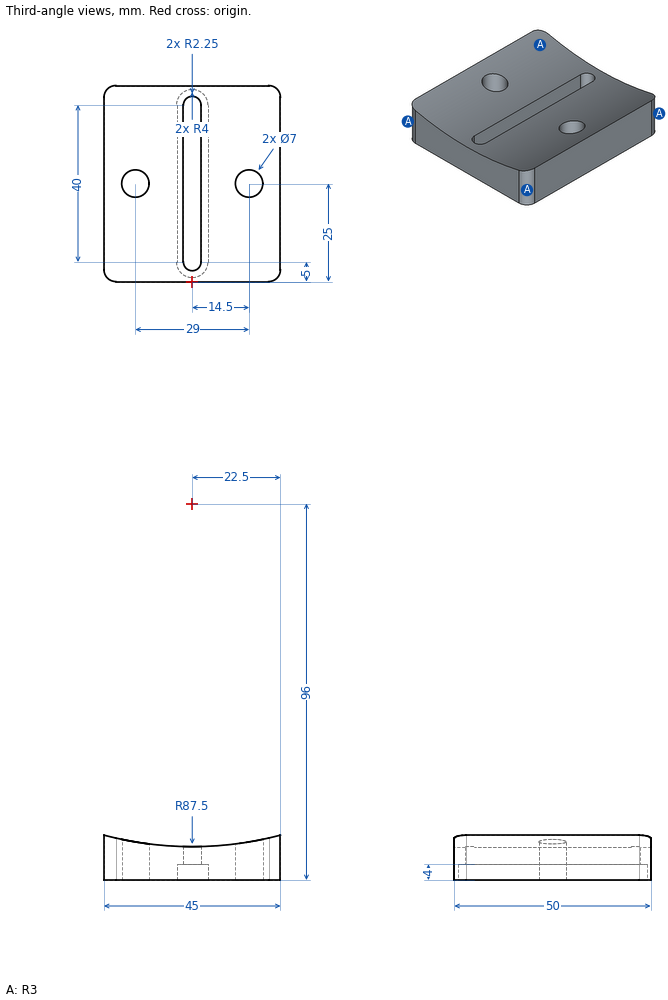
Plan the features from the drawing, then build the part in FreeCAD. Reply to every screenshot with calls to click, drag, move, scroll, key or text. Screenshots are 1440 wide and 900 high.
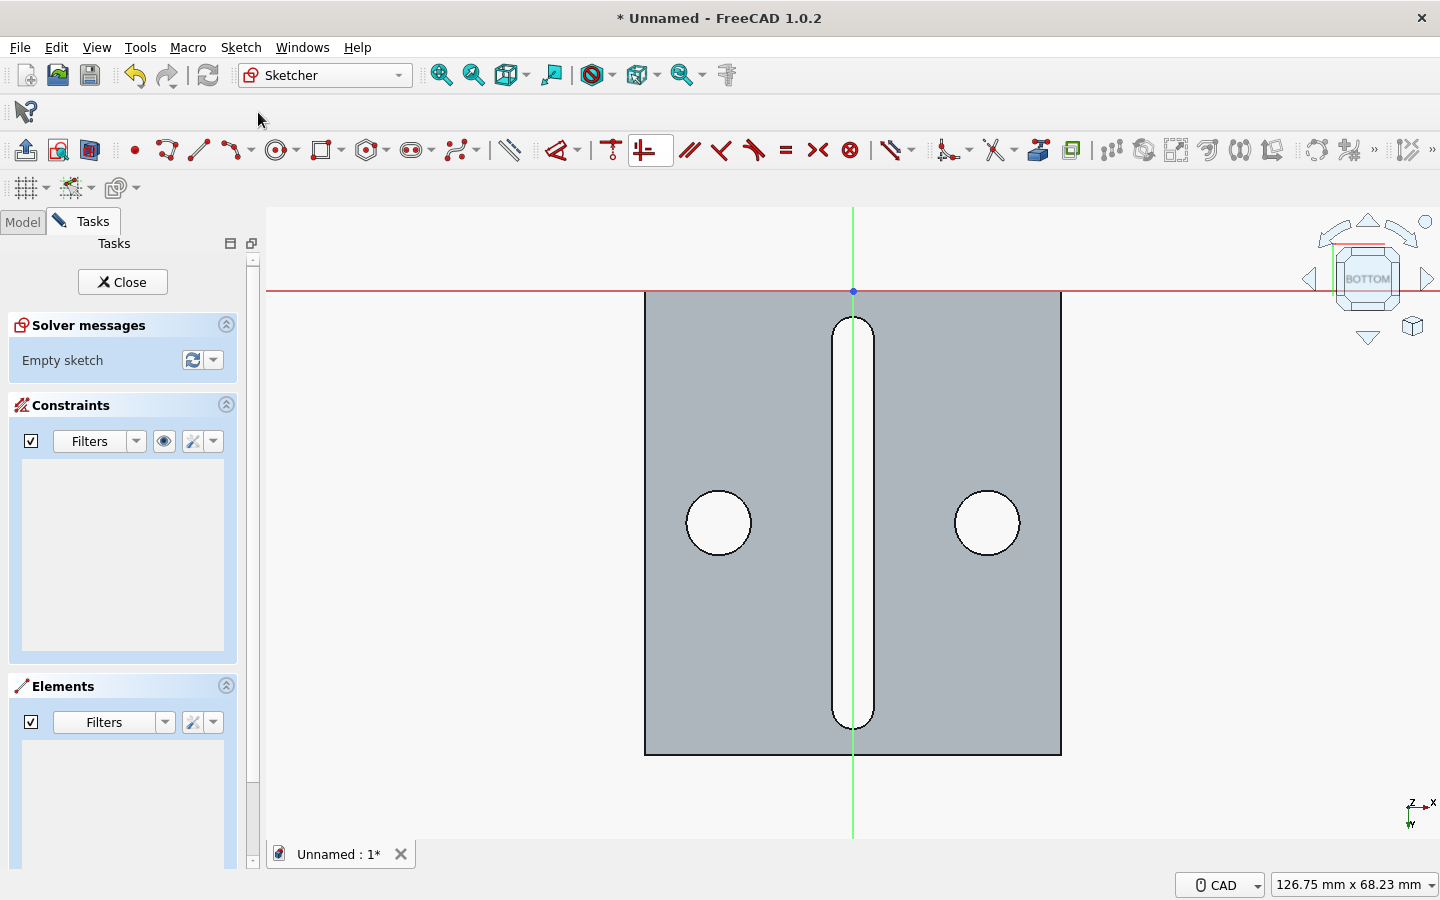
click(412, 150)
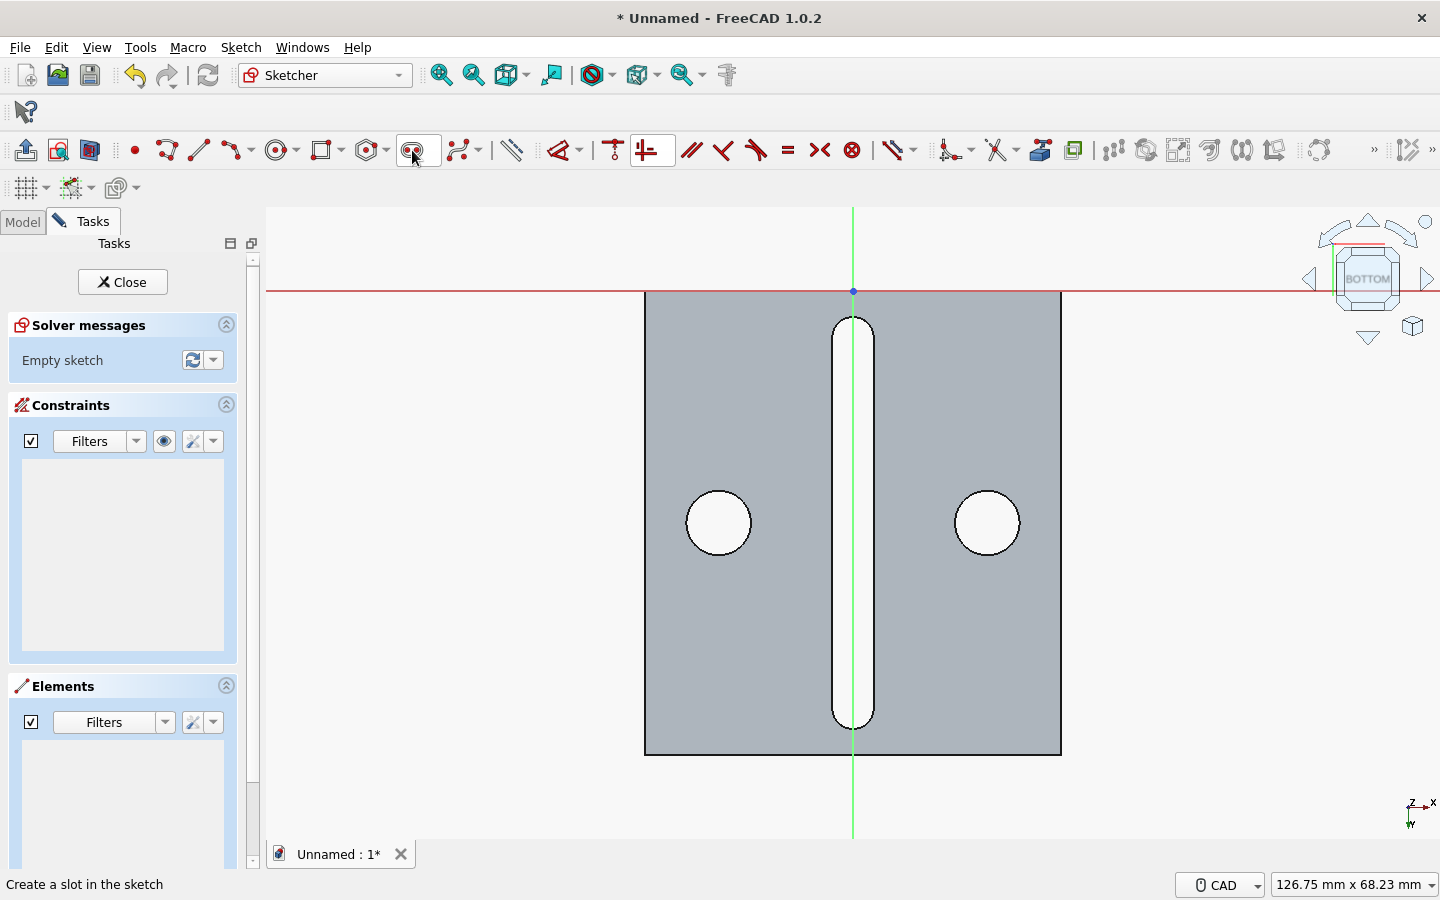
click(853, 708)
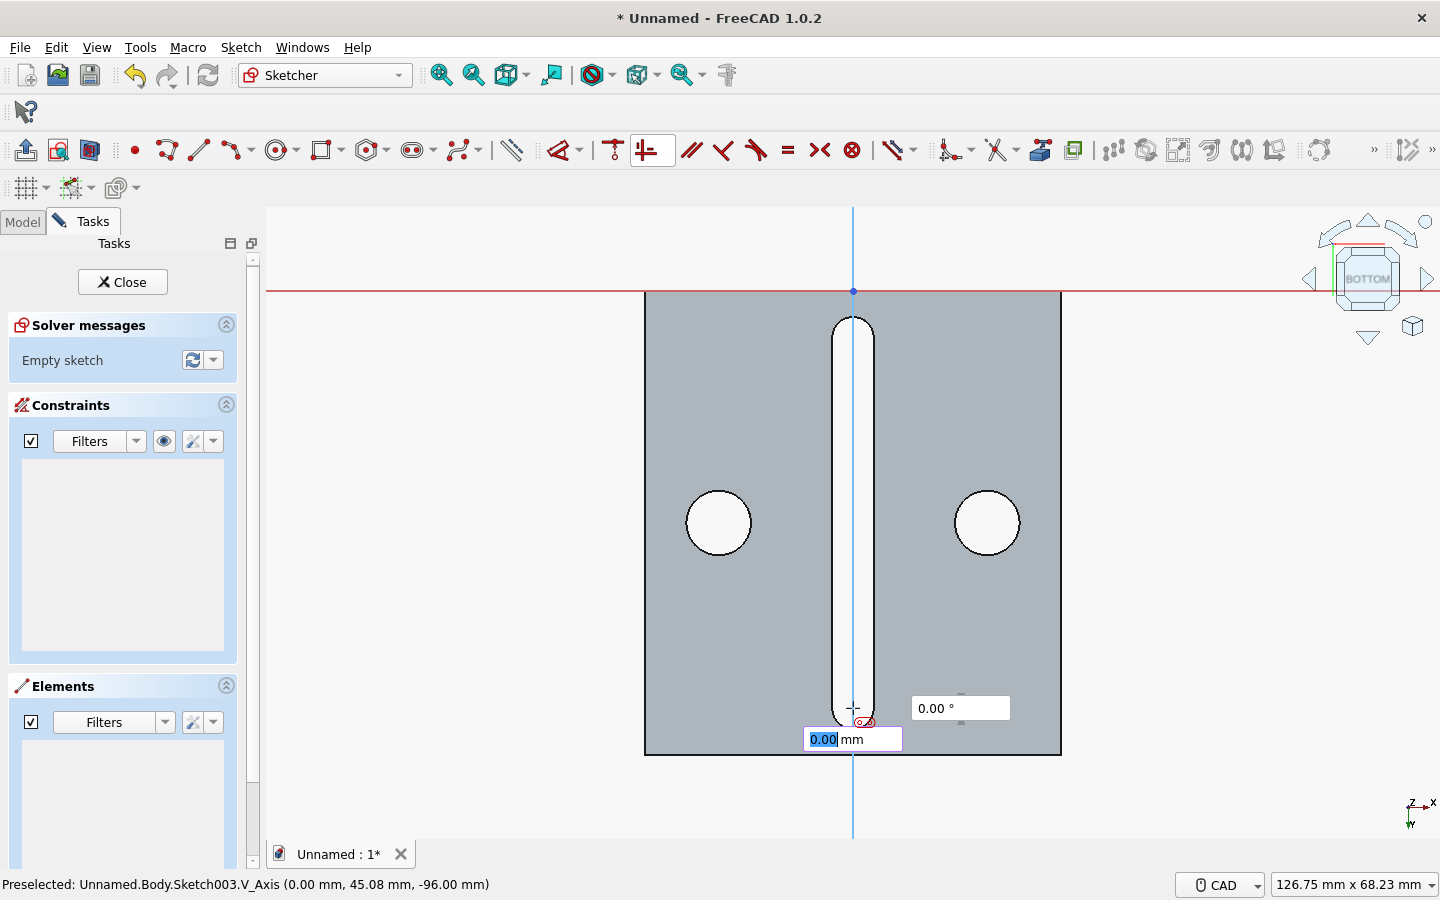
click(862, 338)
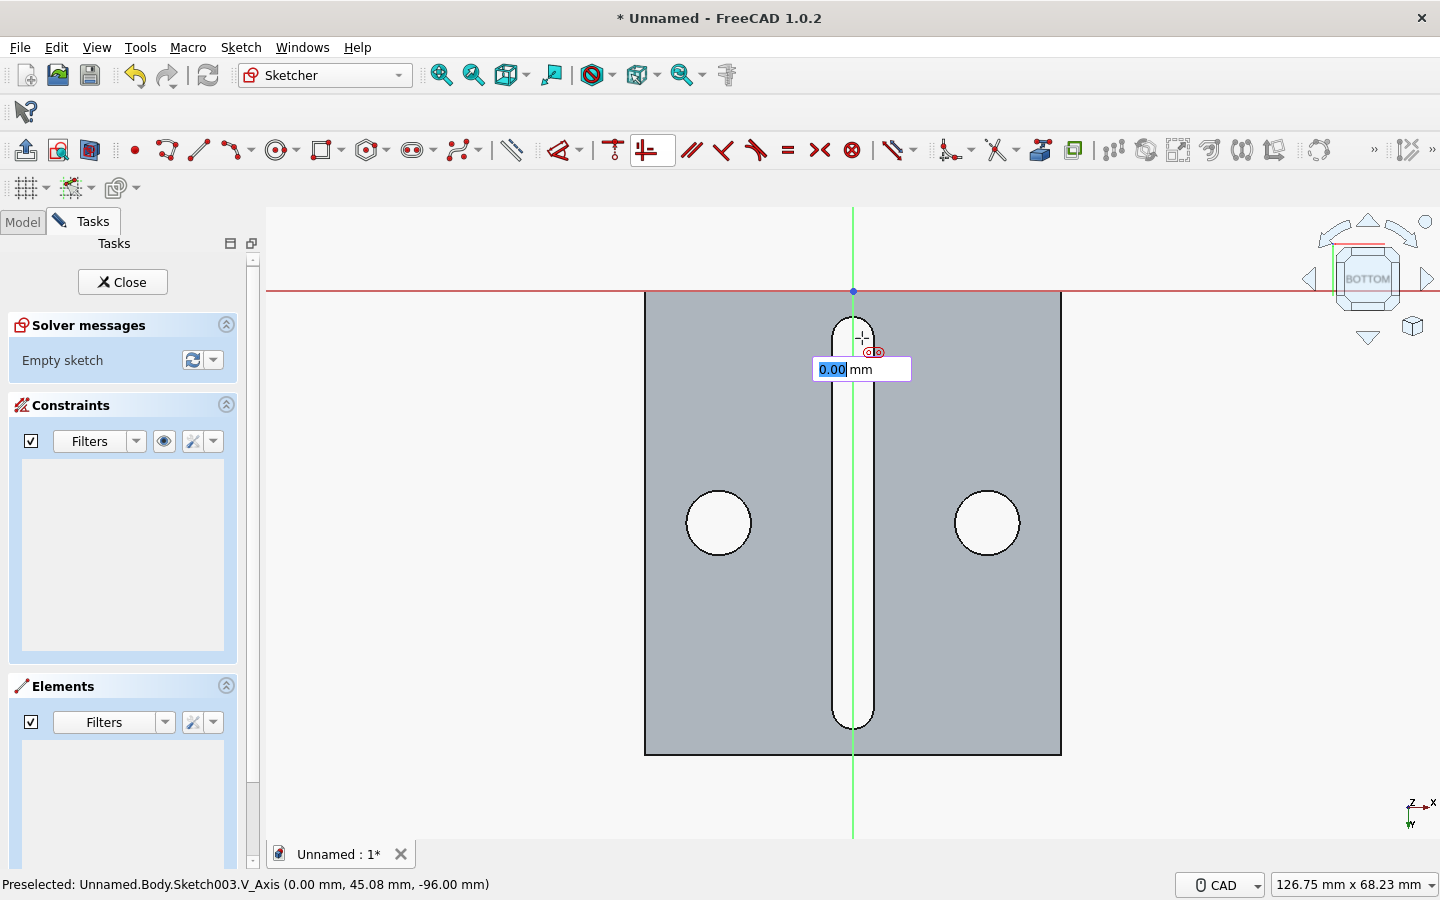
click(816, 523)
key(Escape)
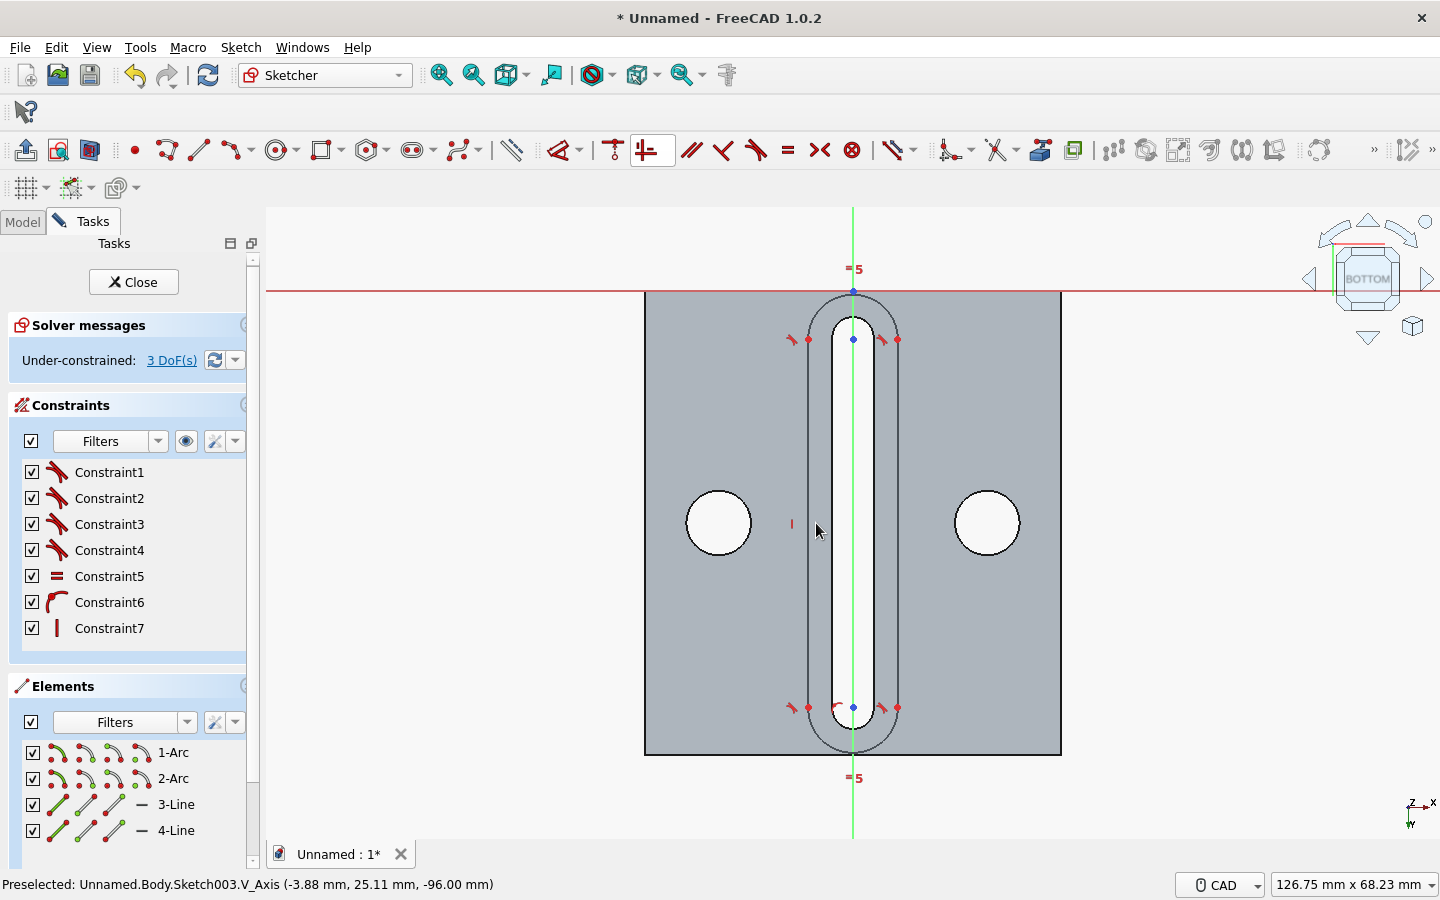
key(d)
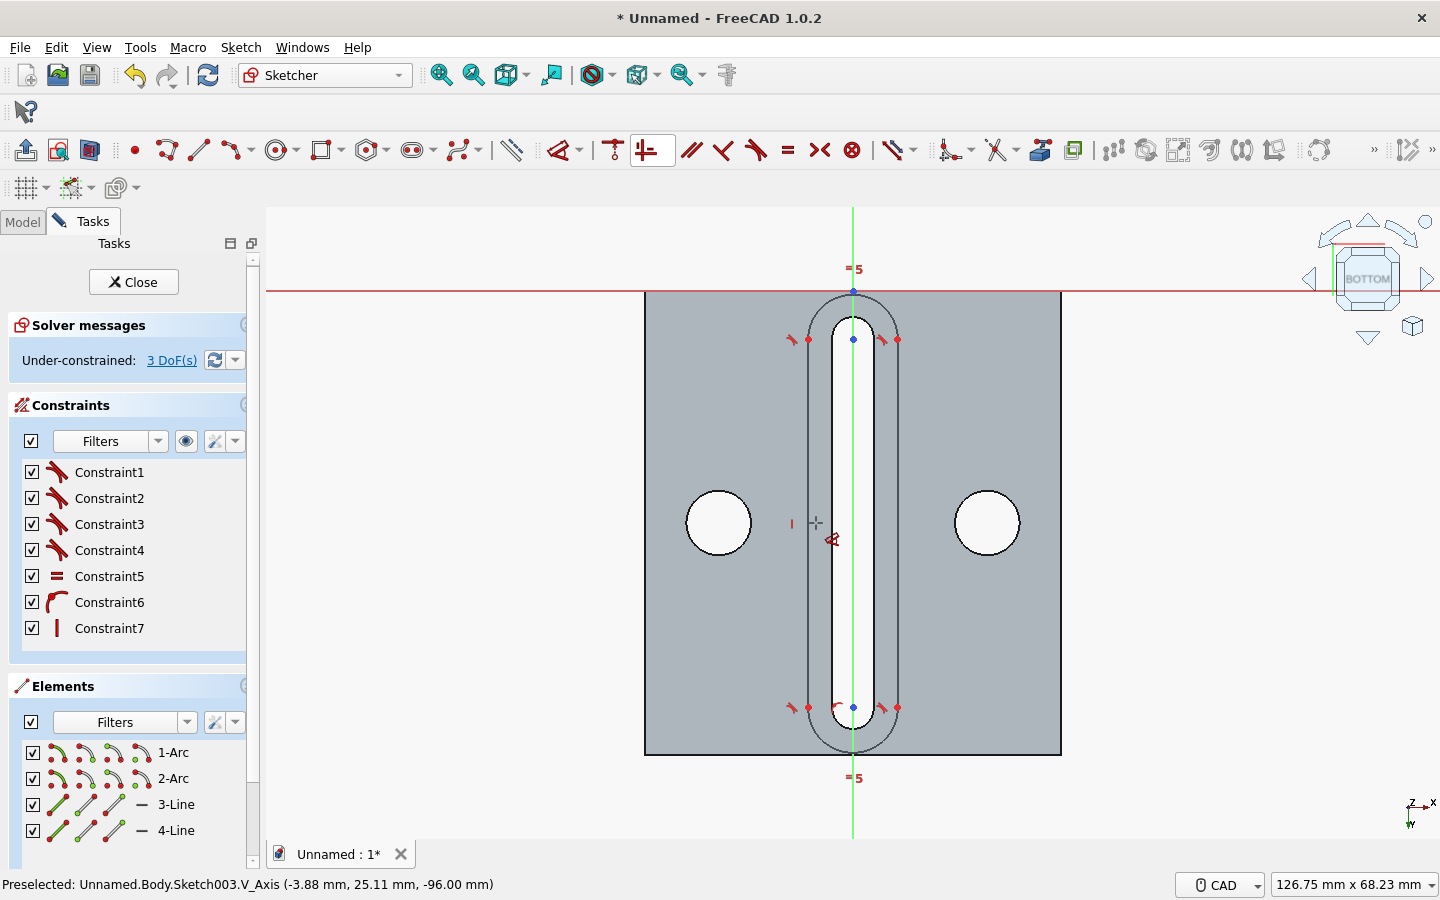
click(827, 744)
click(808, 770)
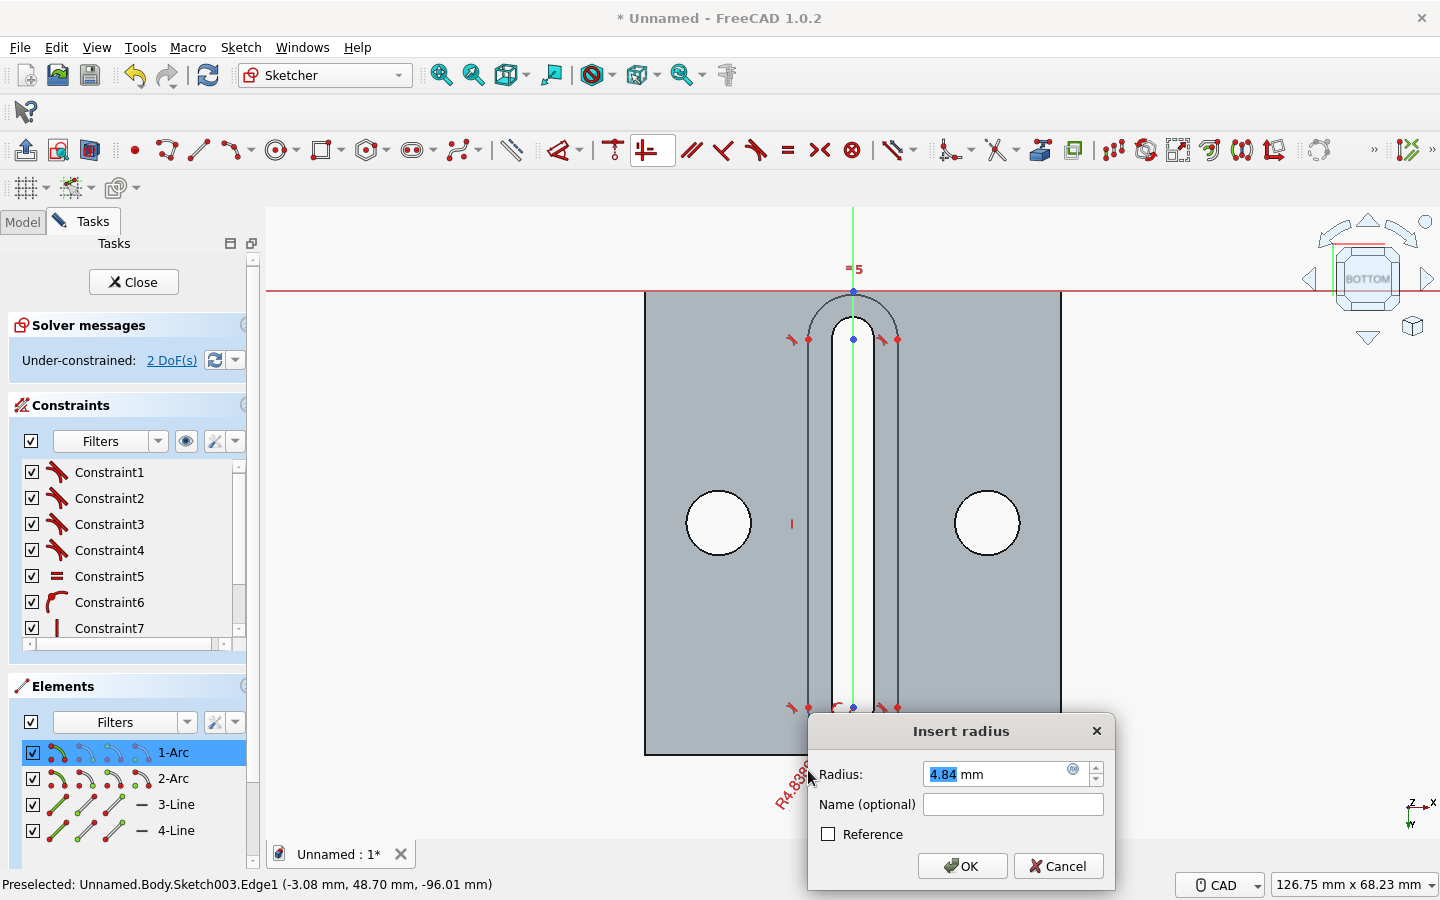
text(4)
key(Return)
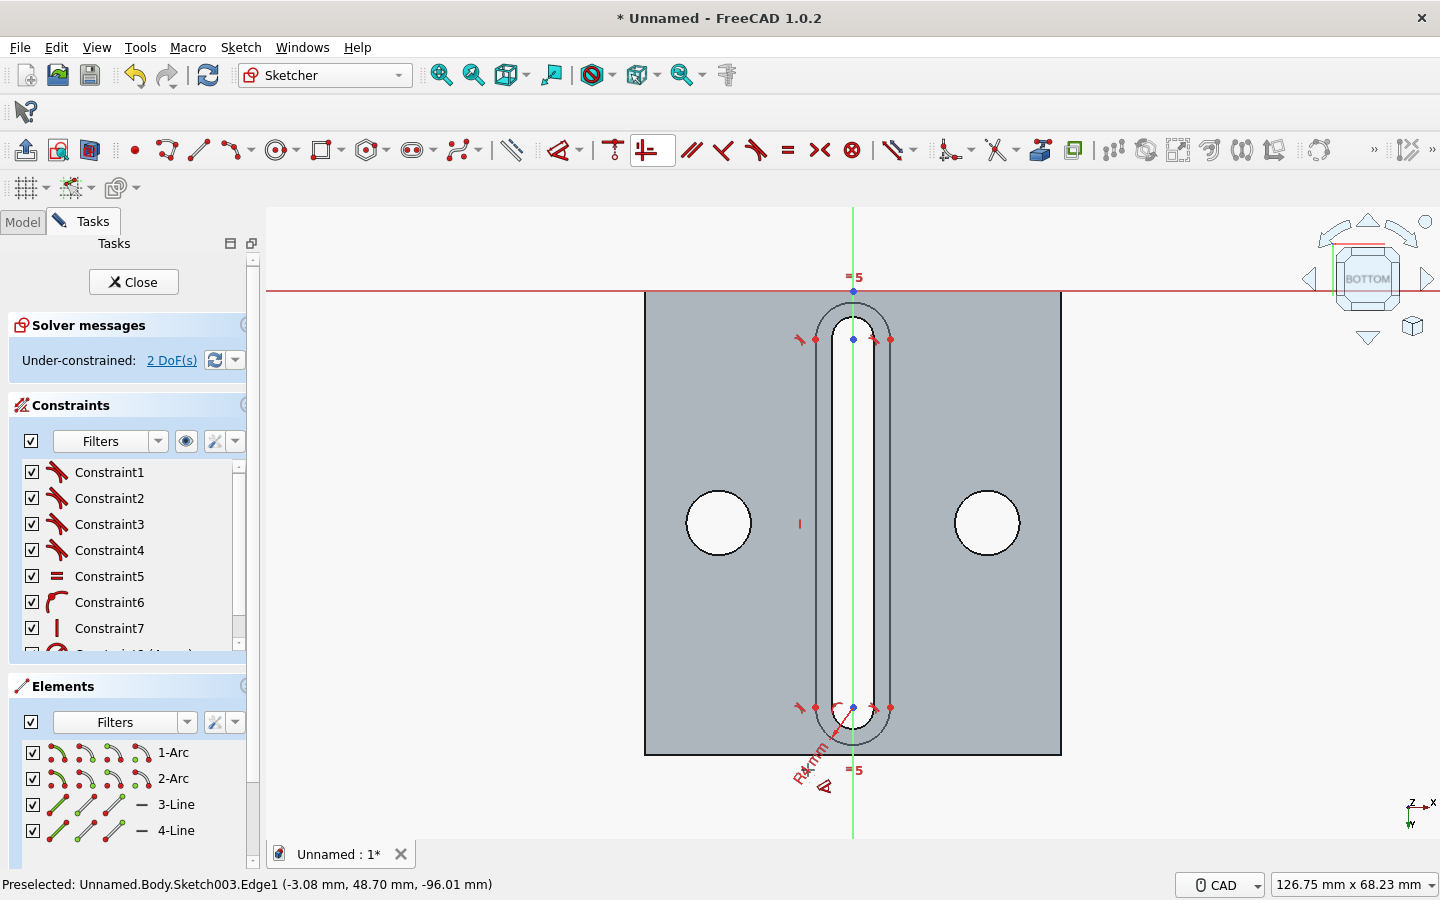
click(816, 597)
click(782, 524)